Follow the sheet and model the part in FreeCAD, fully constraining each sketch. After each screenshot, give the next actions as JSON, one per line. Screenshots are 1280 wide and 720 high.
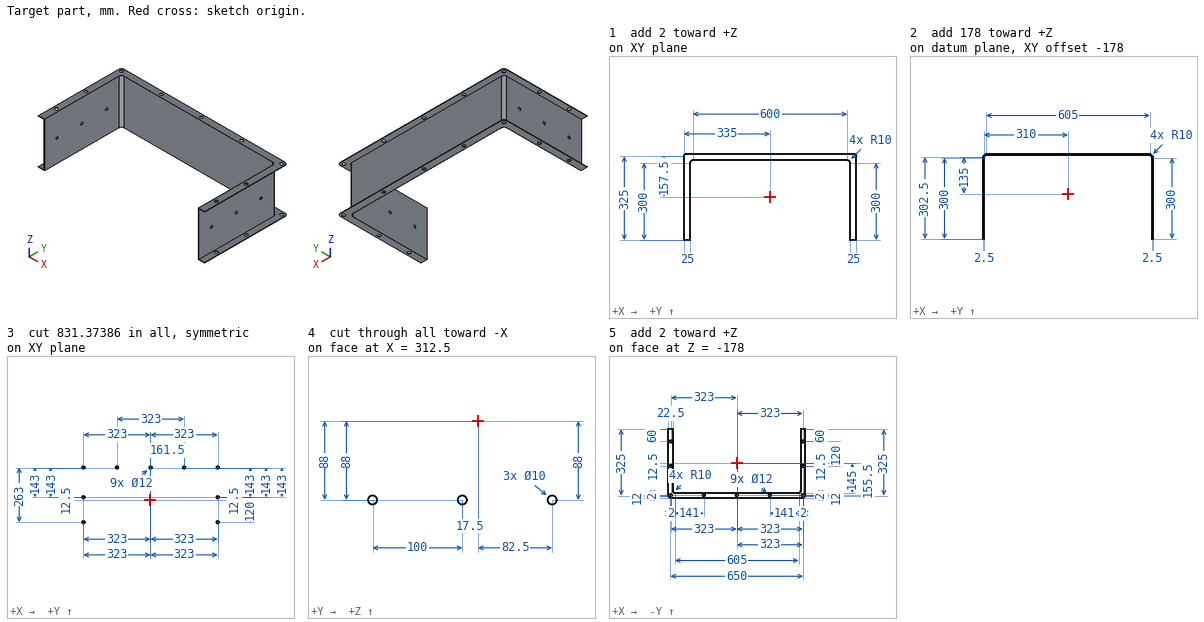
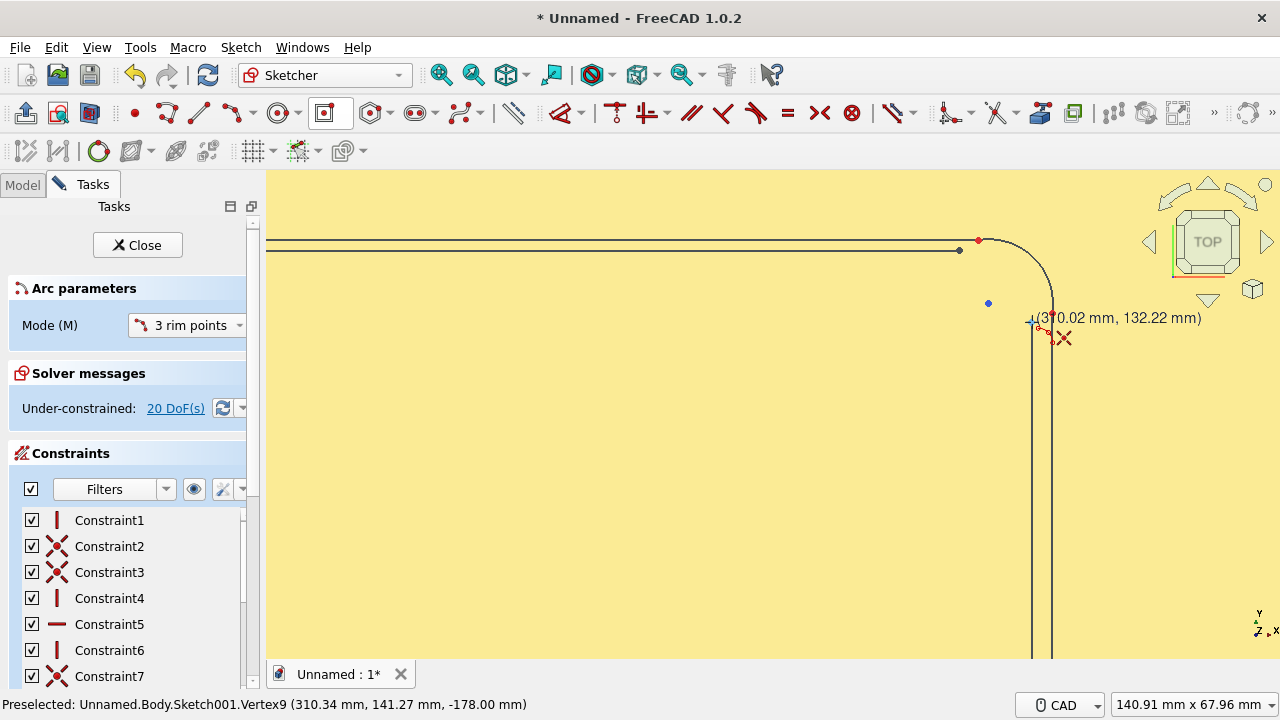
{"action": "left_click", "coordinate": [1032, 323]}
{"action": "left_click", "coordinate": [960, 251]}
{"action": "left_click", "coordinate": [1010, 270]}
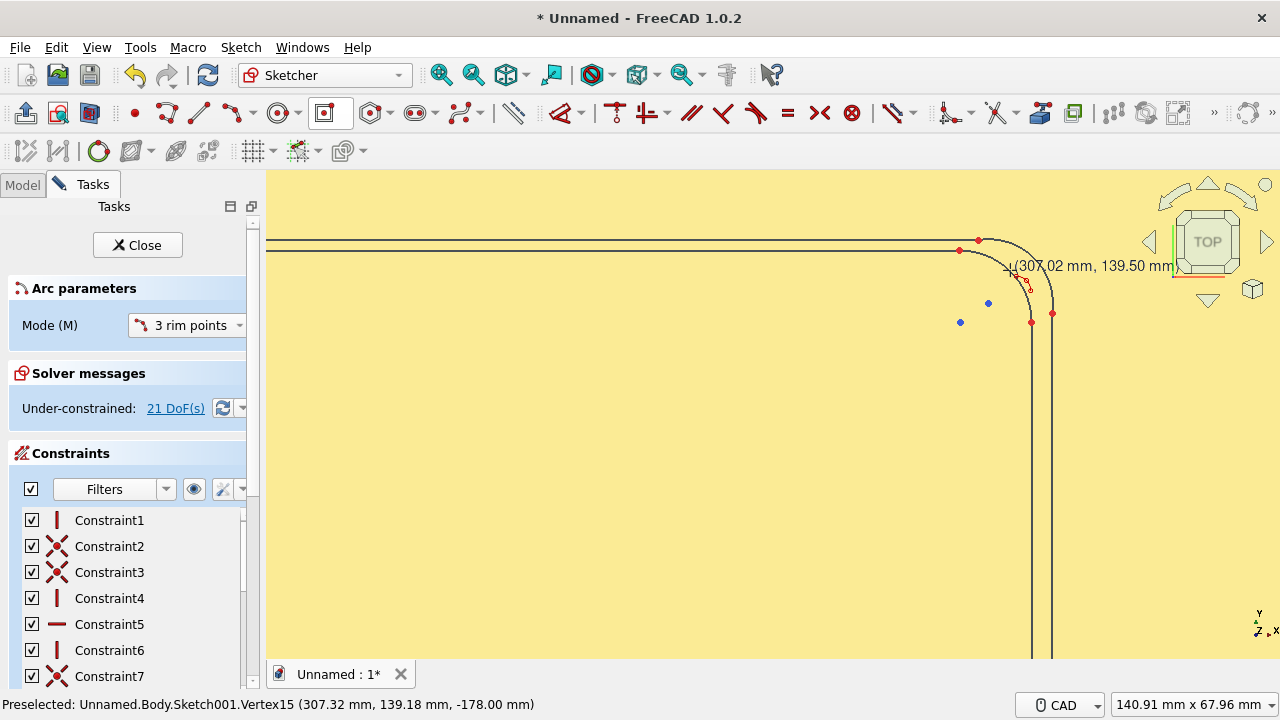
{"action": "scroll", "coordinate": [1002, 267], "scroll_direction": "down", "scroll_amount": 10}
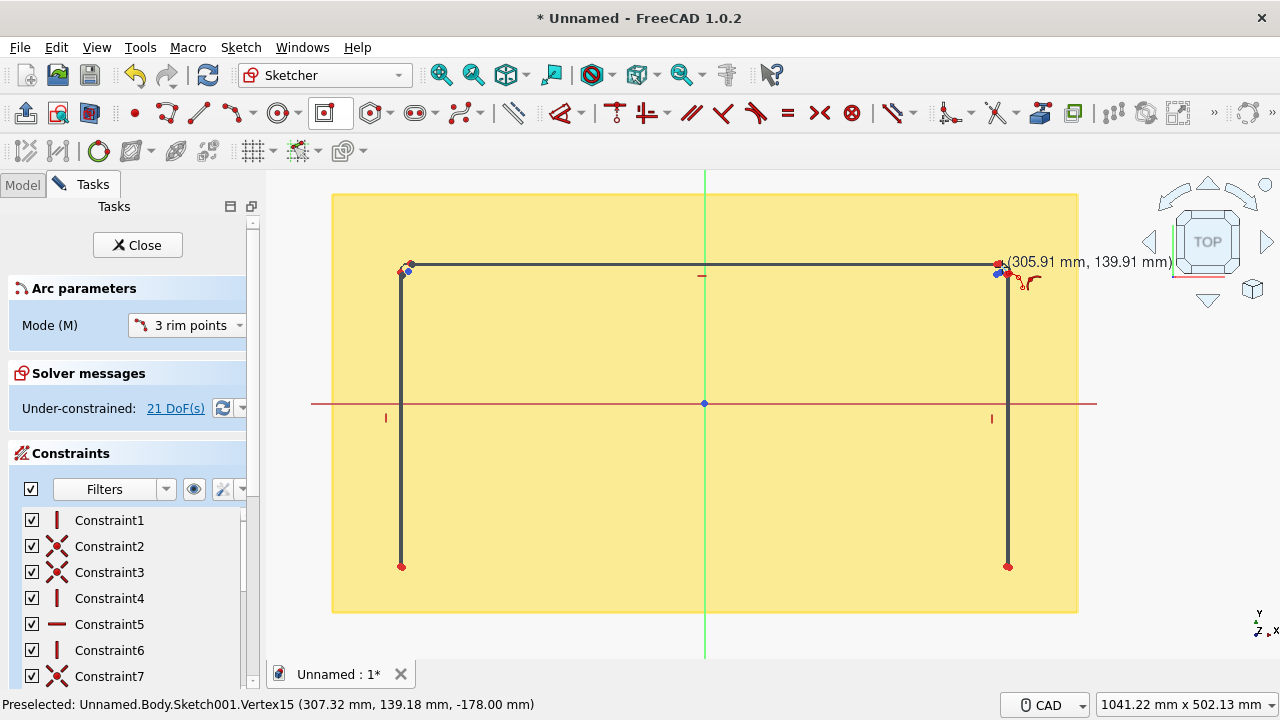
{"action": "scroll", "coordinate": [413, 265], "scroll_direction": "up", "scroll_amount": 10}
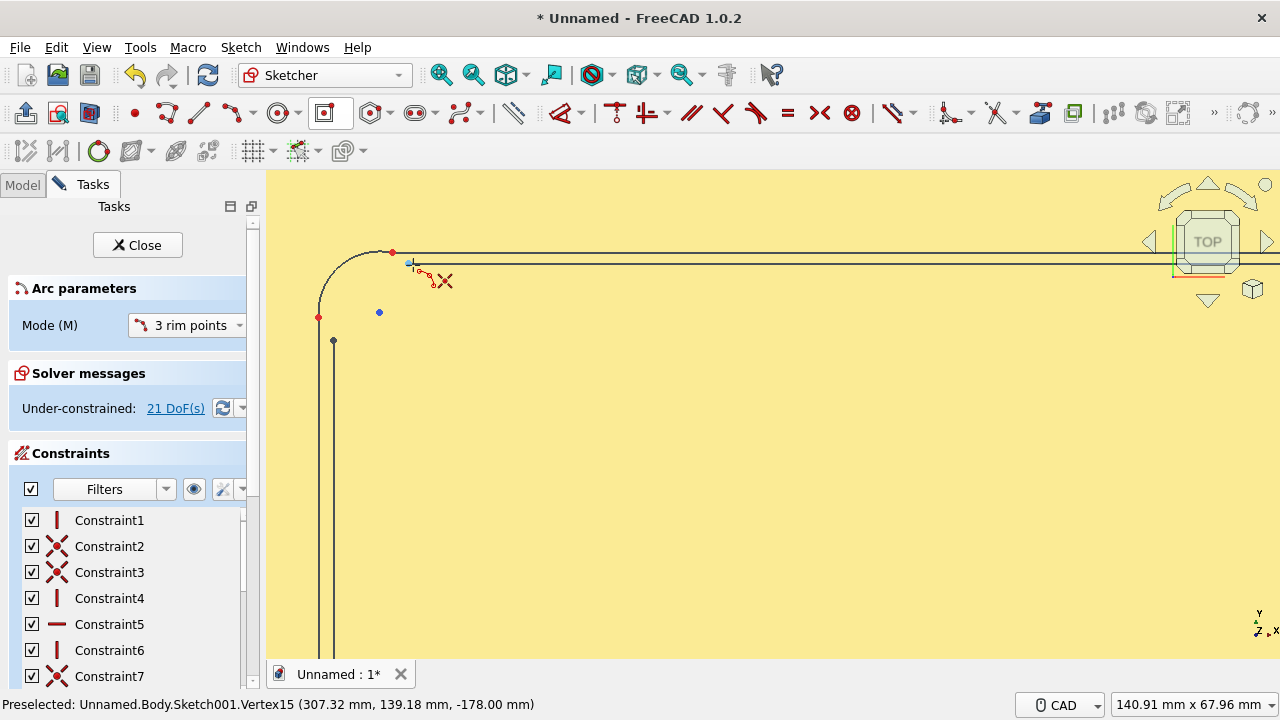
{"action": "left_click", "coordinate": [409, 264]}
{"action": "left_click", "coordinate": [334, 341]}
{"action": "left_click", "coordinate": [358, 283]}
{"action": "key", "text": "Escape"}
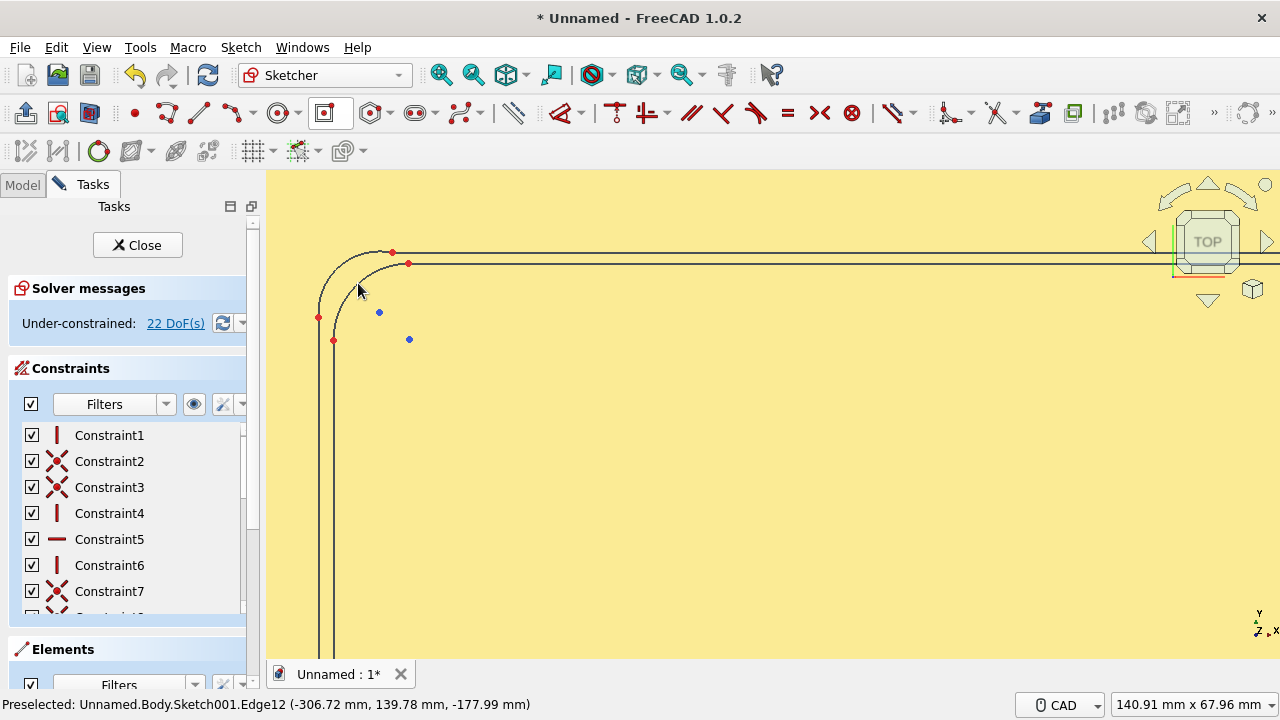
{"action": "scroll", "coordinate": [413, 265], "scroll_direction": "down", "scroll_amount": 10}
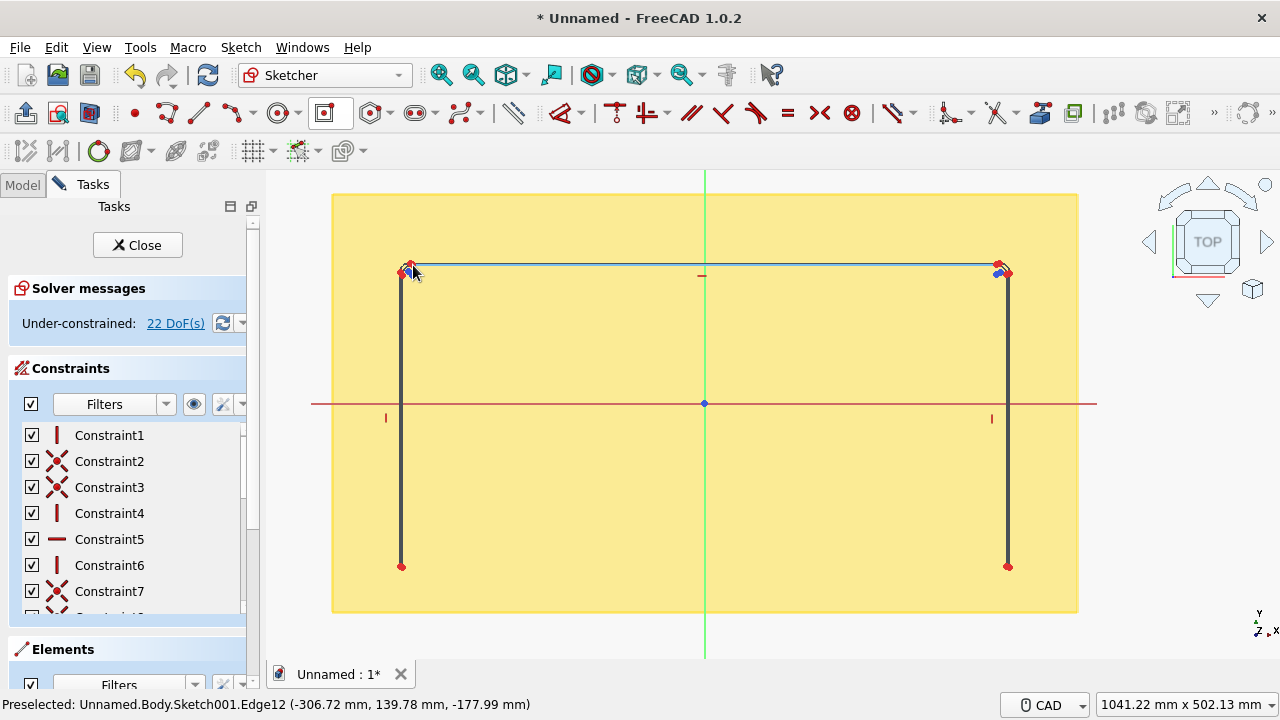
{"action": "scroll", "coordinate": [402, 363], "scroll_direction": "up", "scroll_amount": 10}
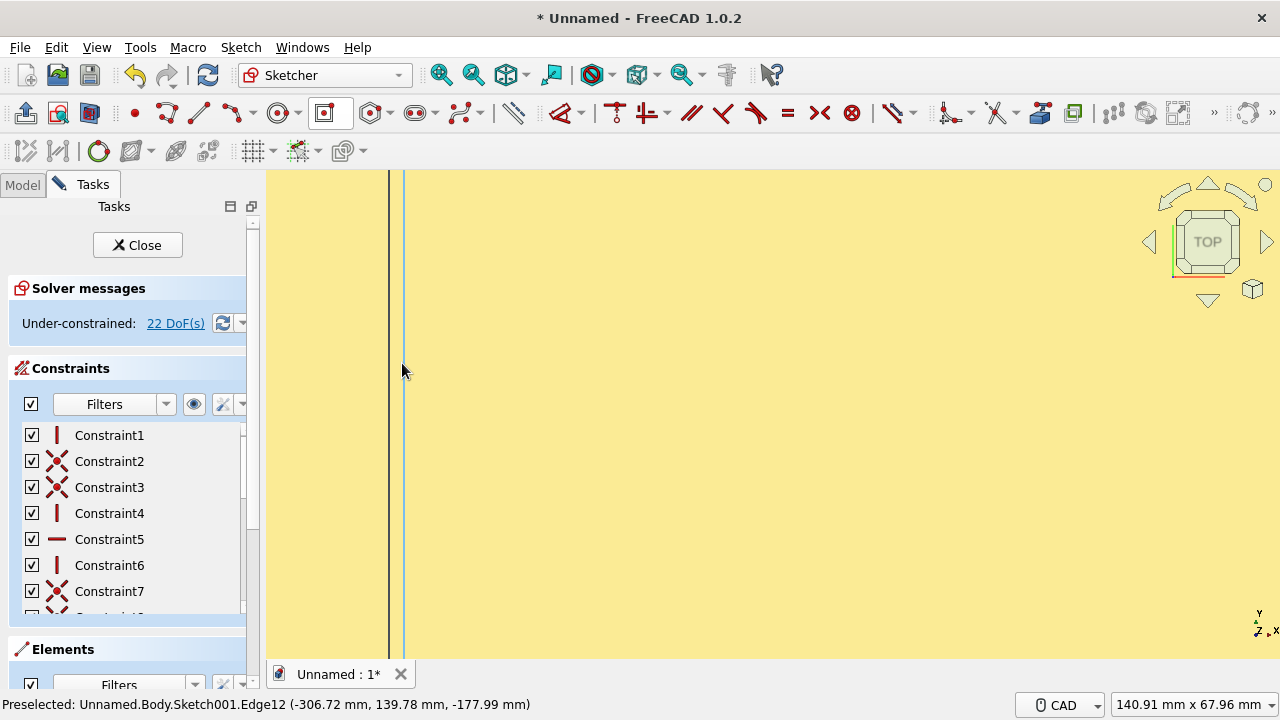
{"action": "left_click", "coordinate": [404, 360]}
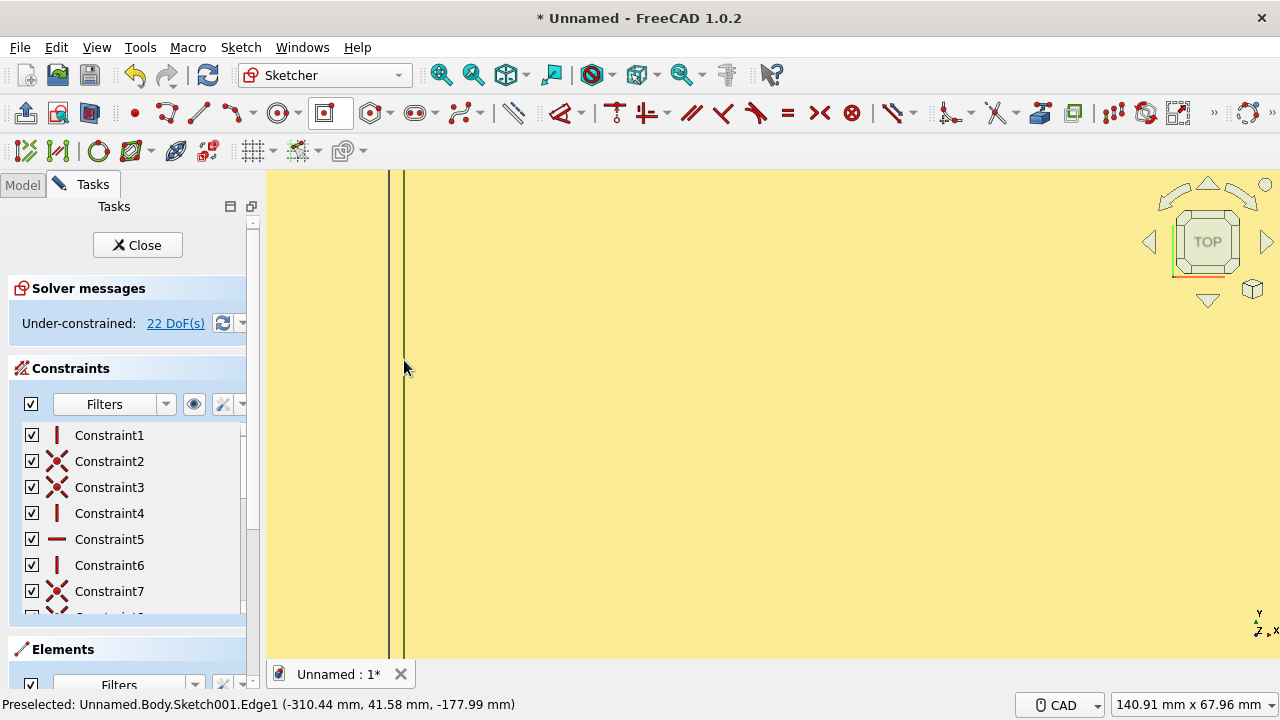
{"action": "scroll", "coordinate": [402, 363], "scroll_direction": "down", "scroll_amount": 10}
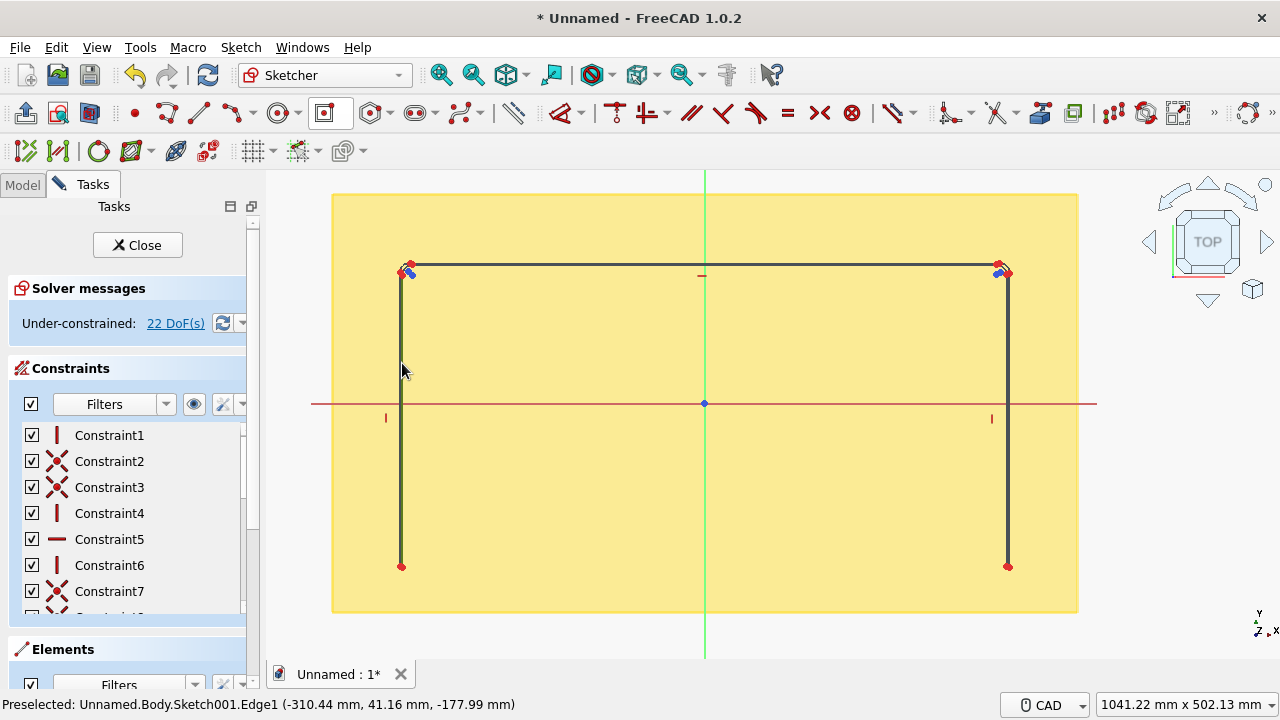
{"action": "scroll", "coordinate": [408, 266], "scroll_direction": "up", "scroll_amount": 9}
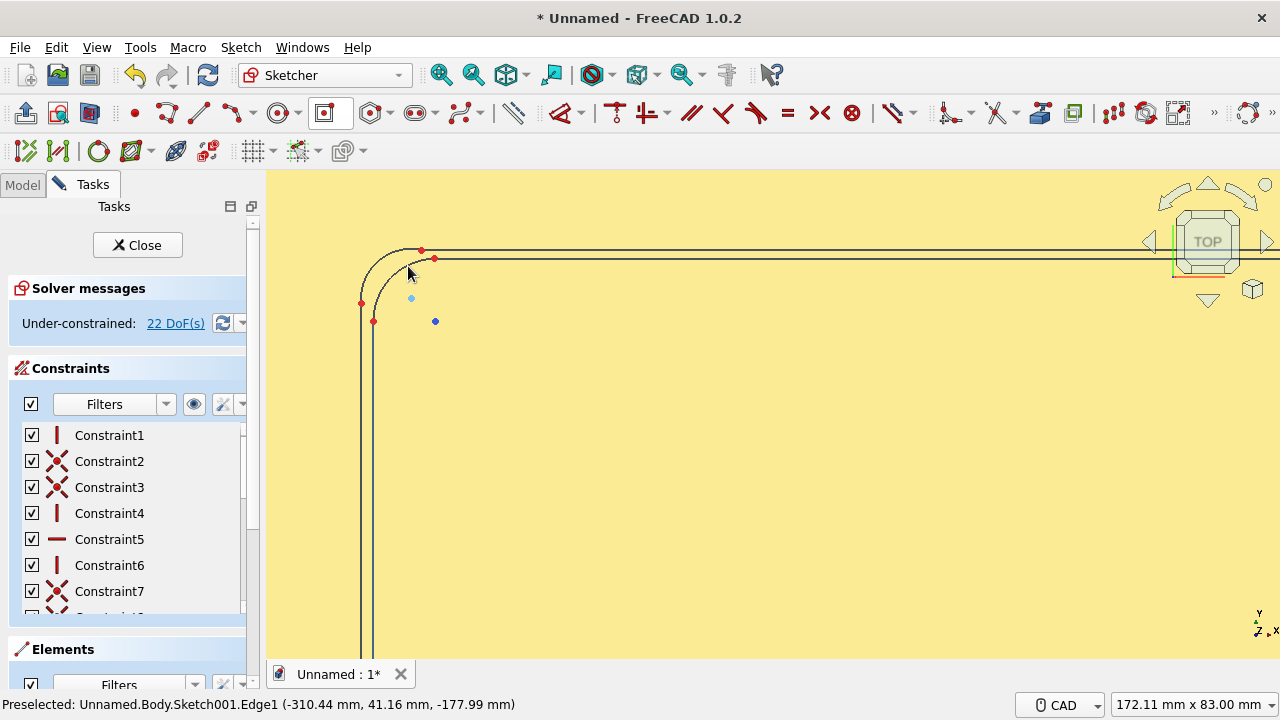
{"action": "left_click", "coordinate": [407, 266]}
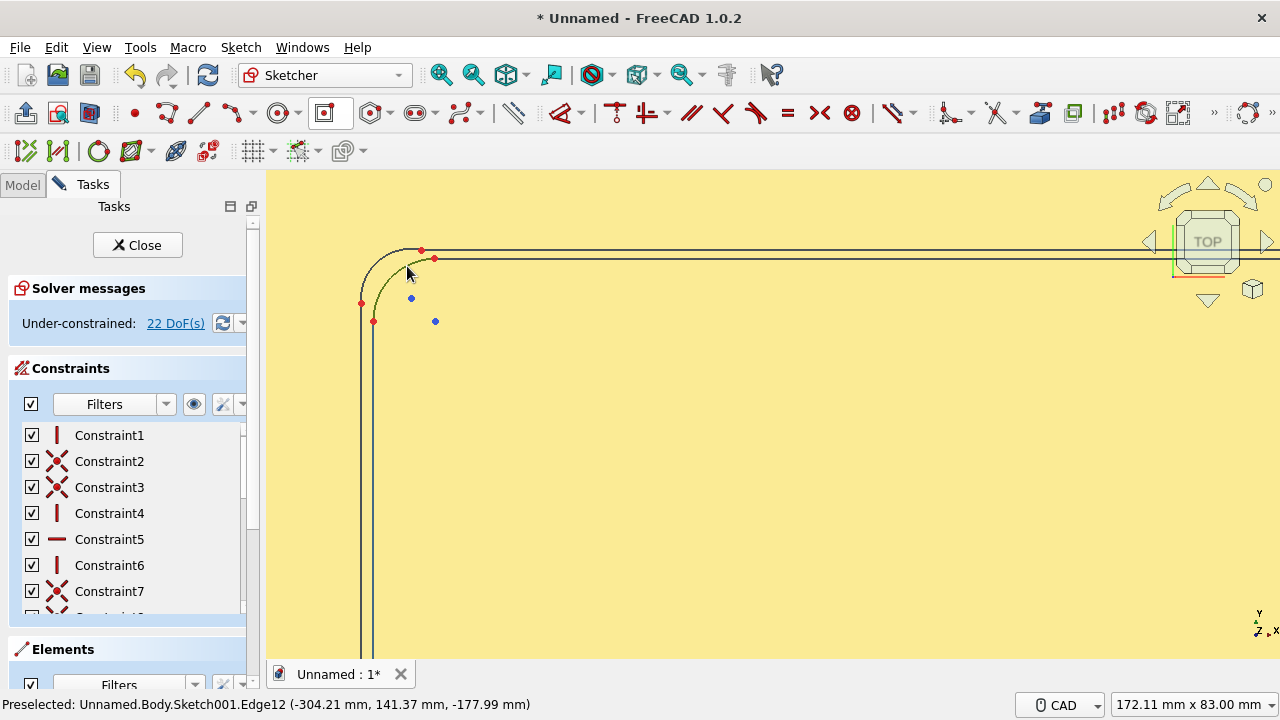
{"action": "left_click", "coordinate": [756, 114]}